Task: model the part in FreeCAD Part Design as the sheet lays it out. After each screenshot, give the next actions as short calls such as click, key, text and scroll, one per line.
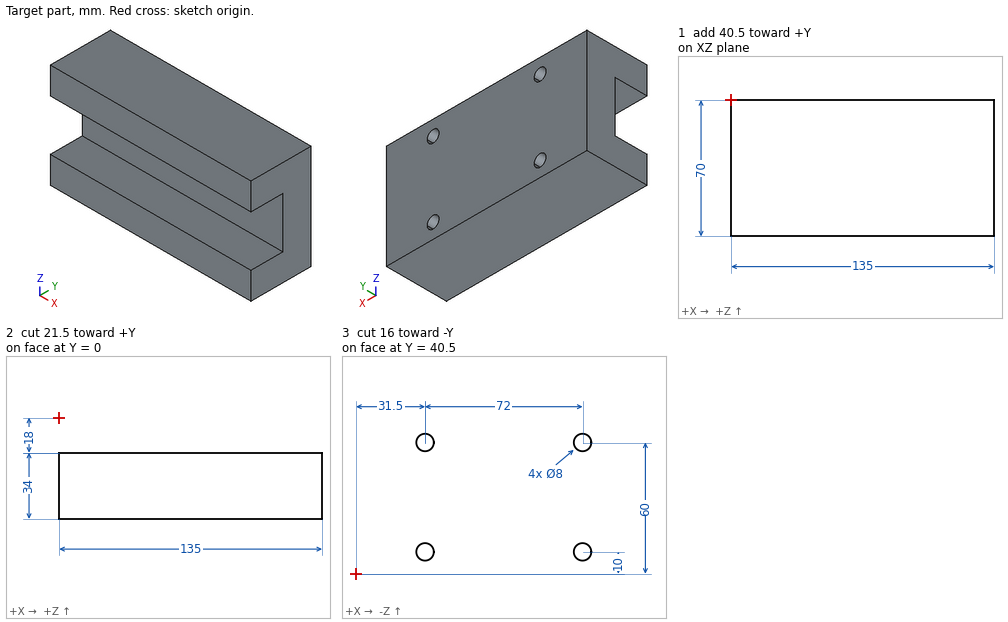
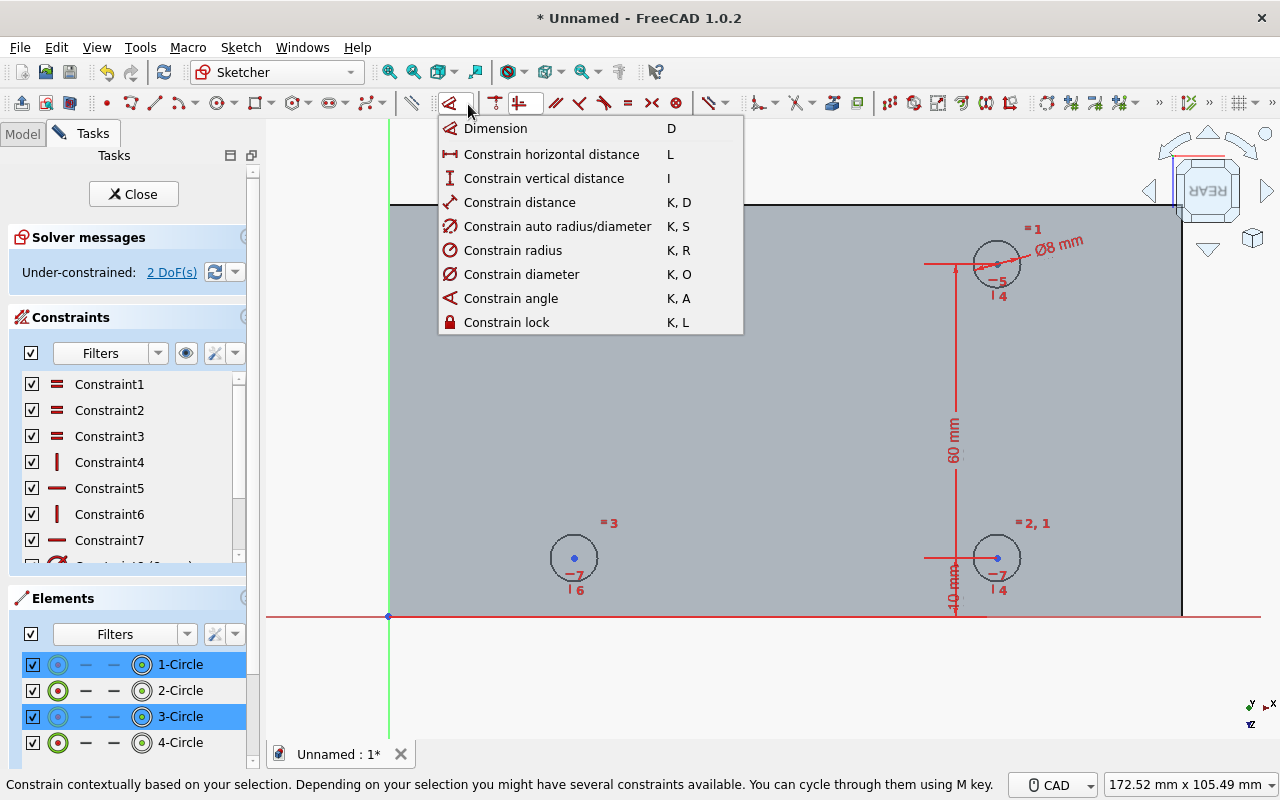
click(591, 154)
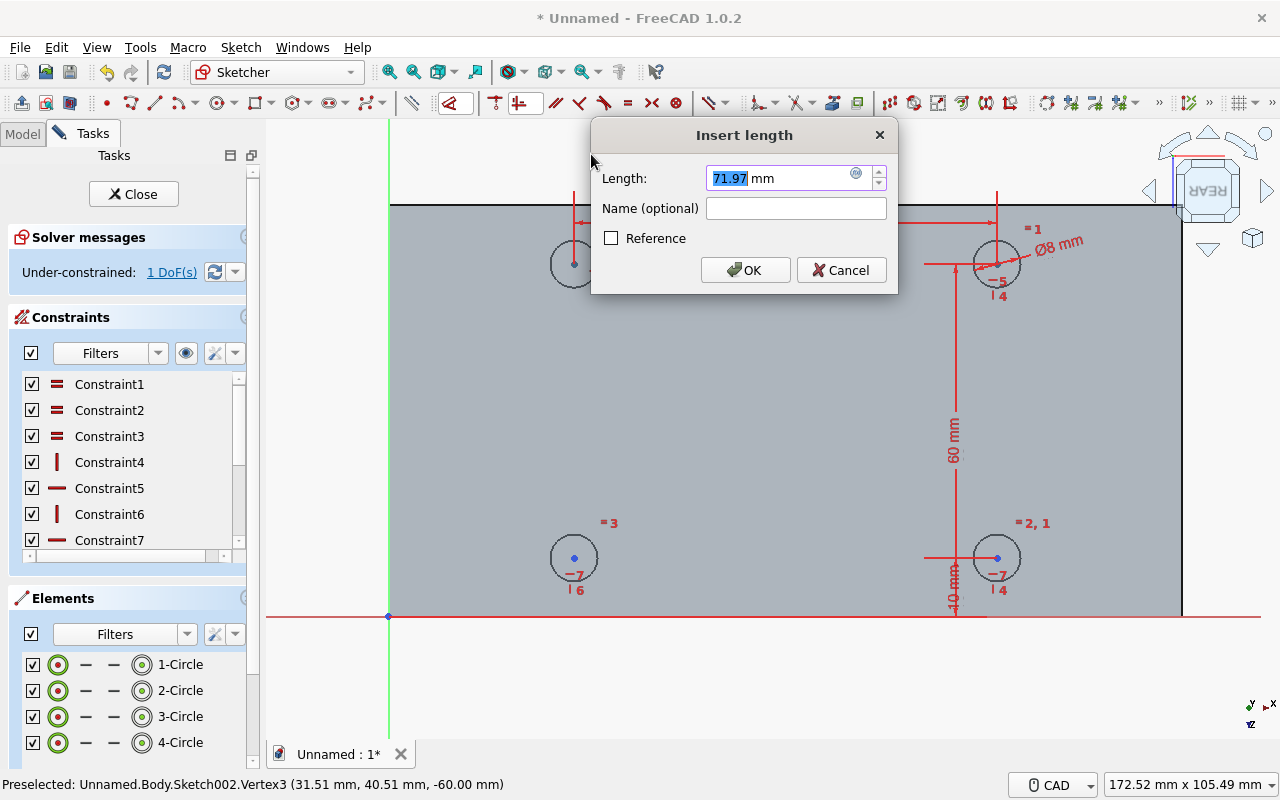
text(72)
key(Return)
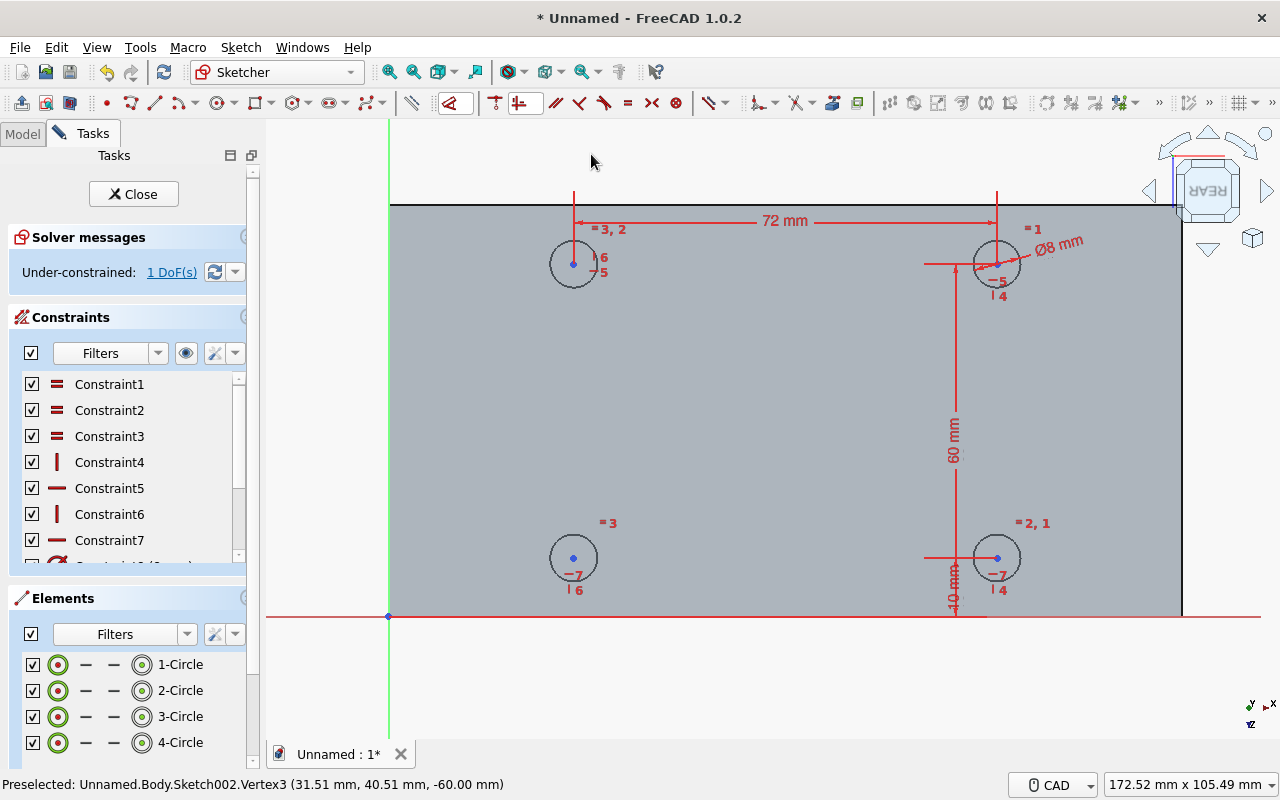
click(574, 264)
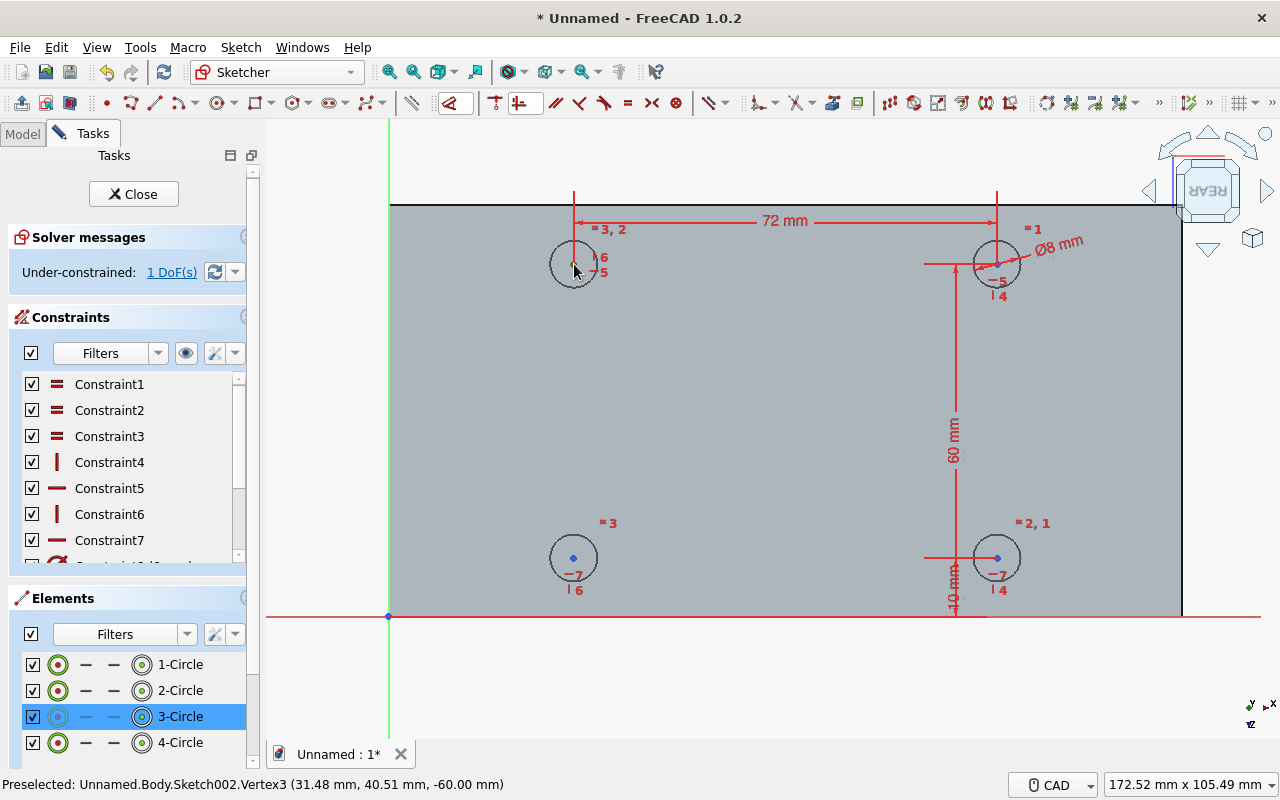
key(l)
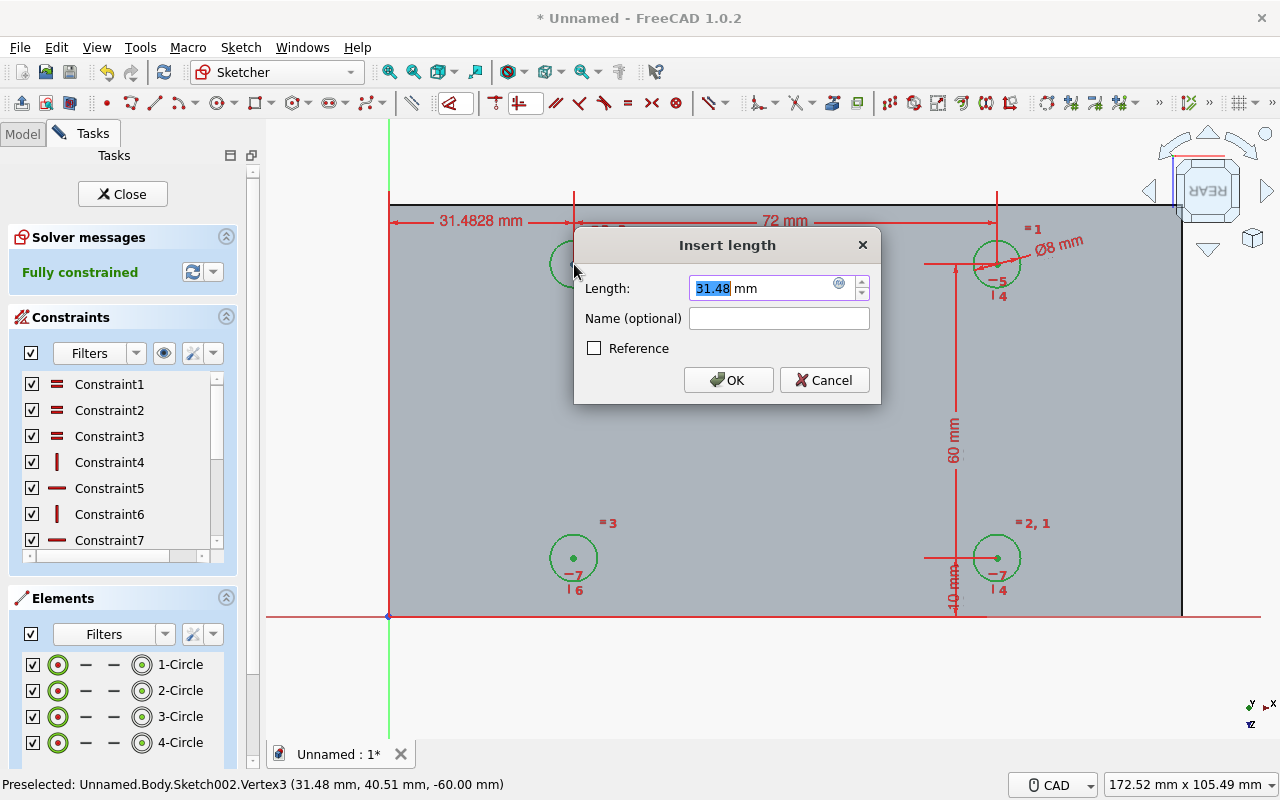
text(31.5)
key(Return)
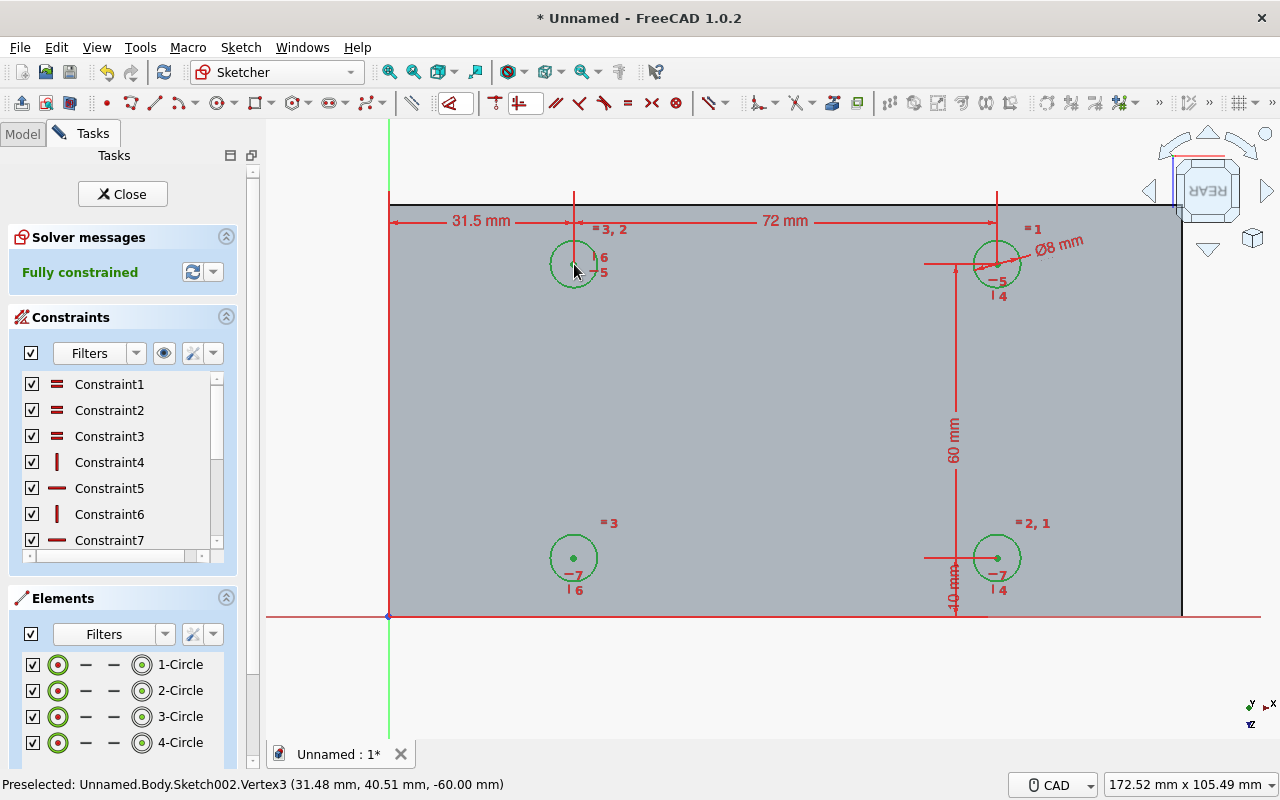
click(123, 194)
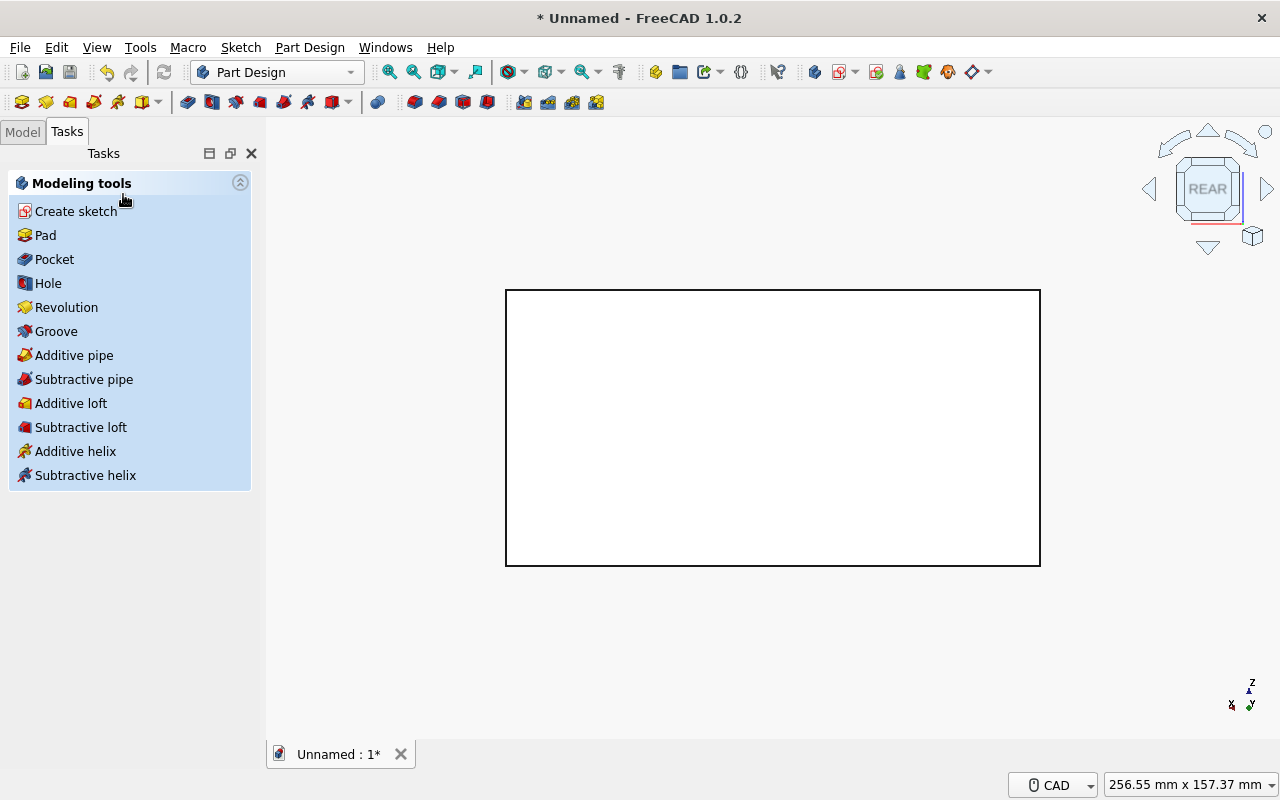
click(188, 102)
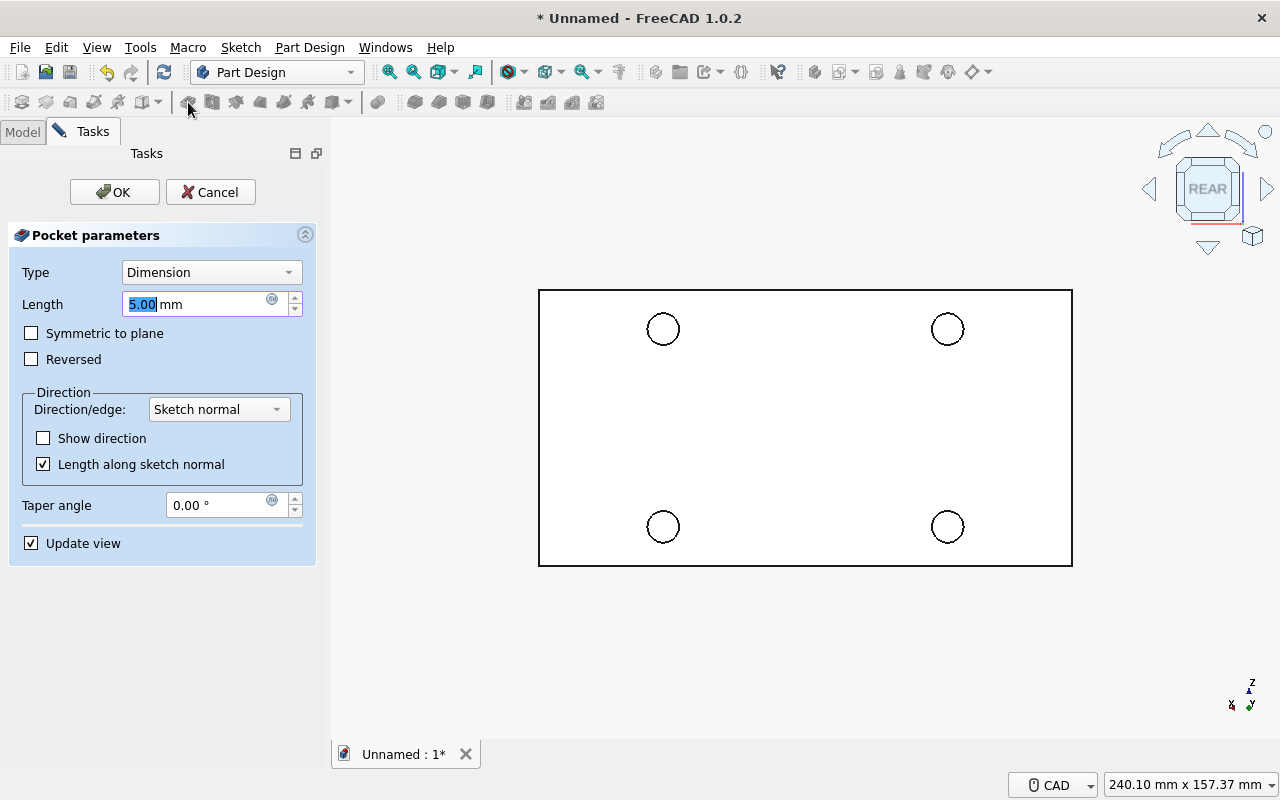
text(16)
key(Tab)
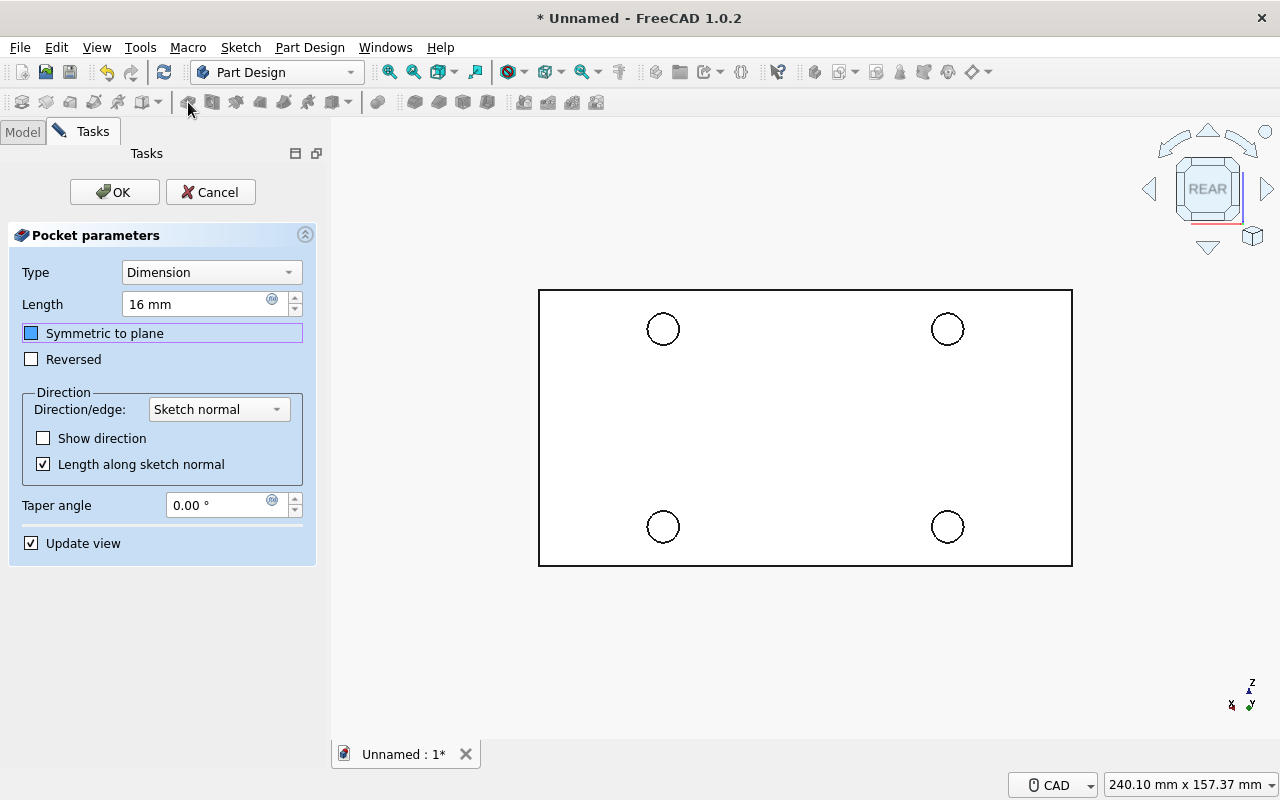
click(115, 192)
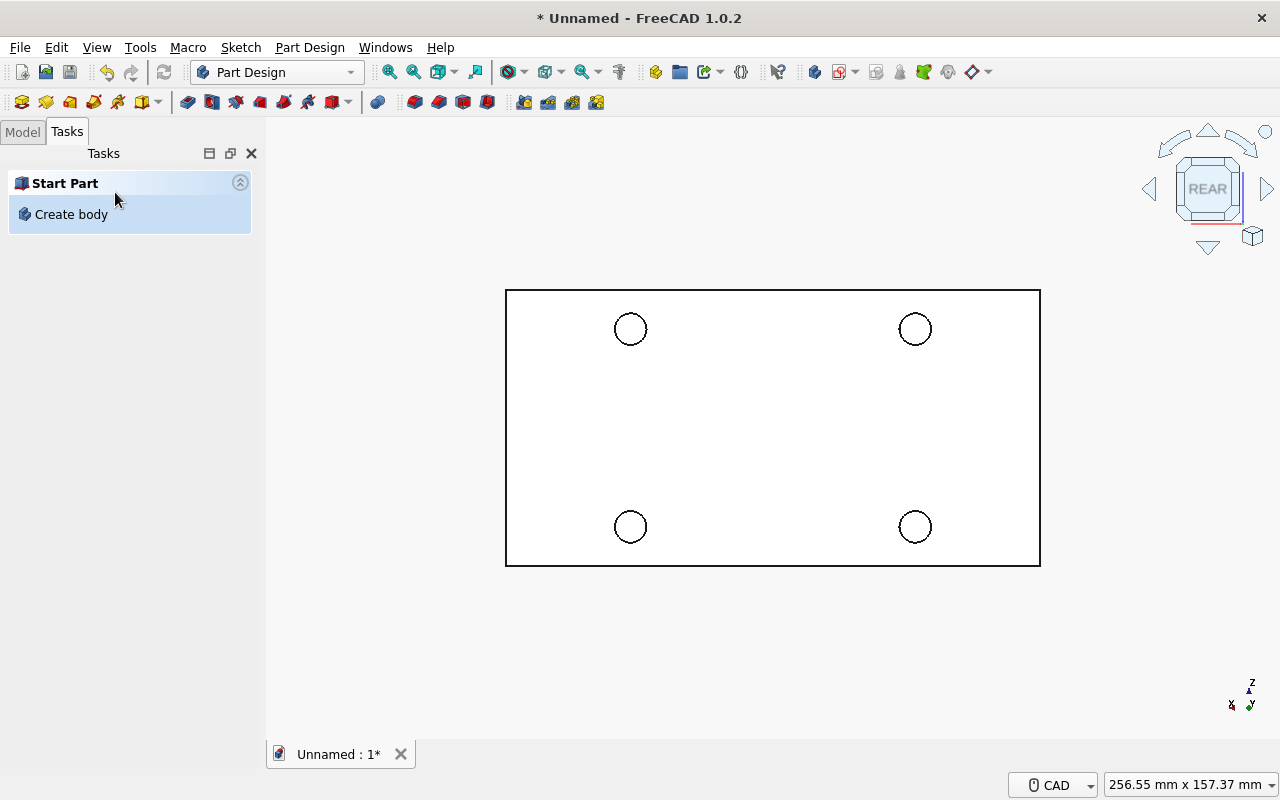
key(0)